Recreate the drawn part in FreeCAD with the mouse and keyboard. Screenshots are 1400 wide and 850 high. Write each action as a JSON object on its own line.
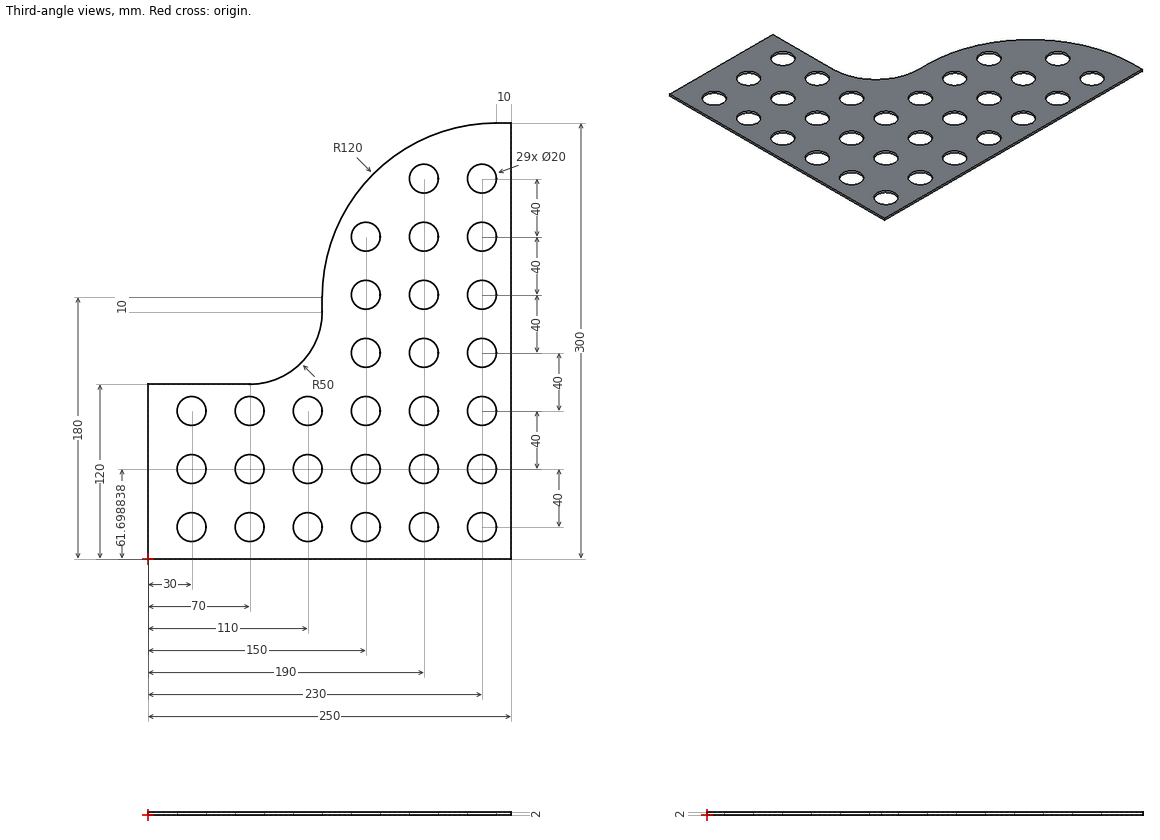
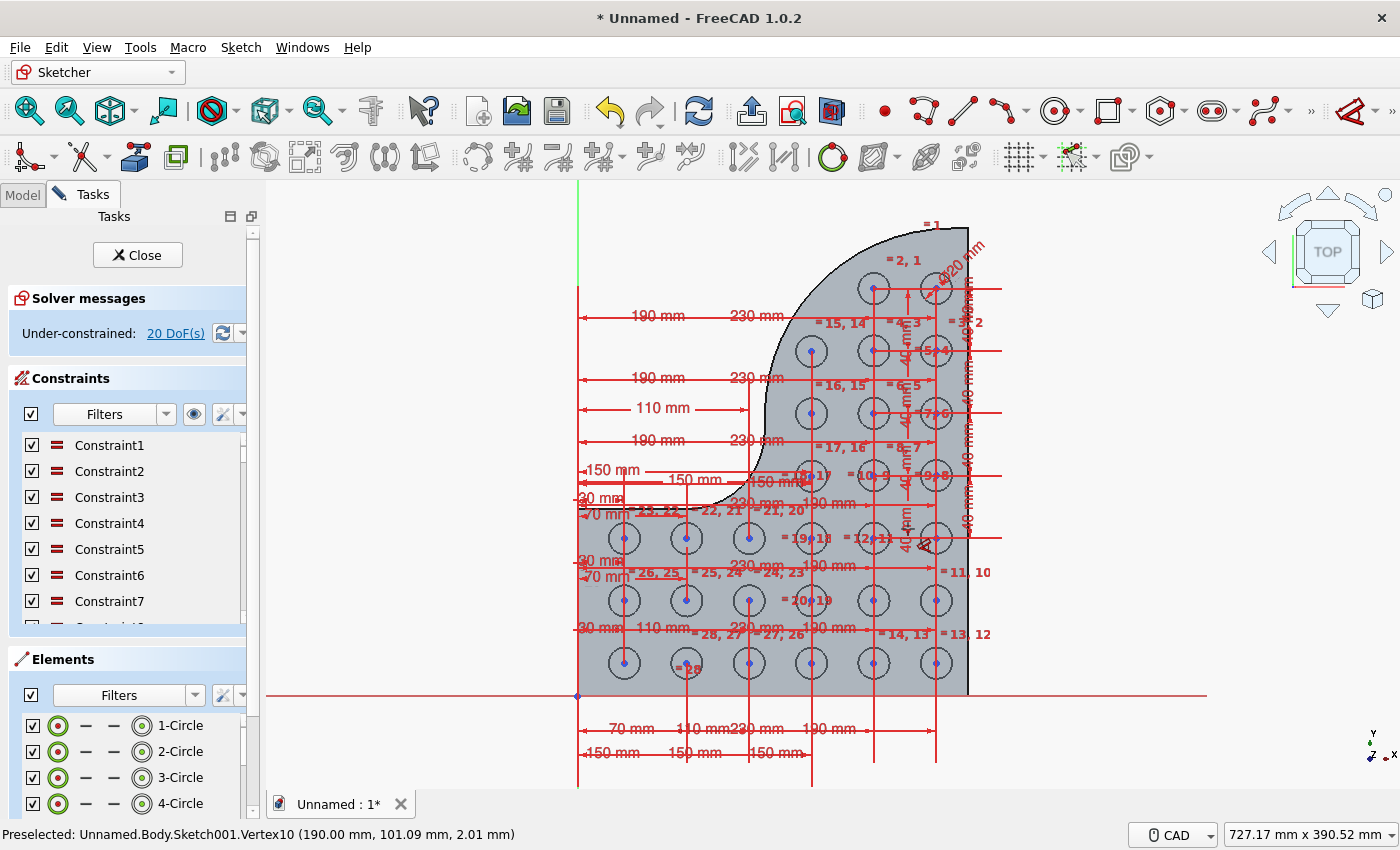
{"action": "left_click", "coordinate": [936, 538]}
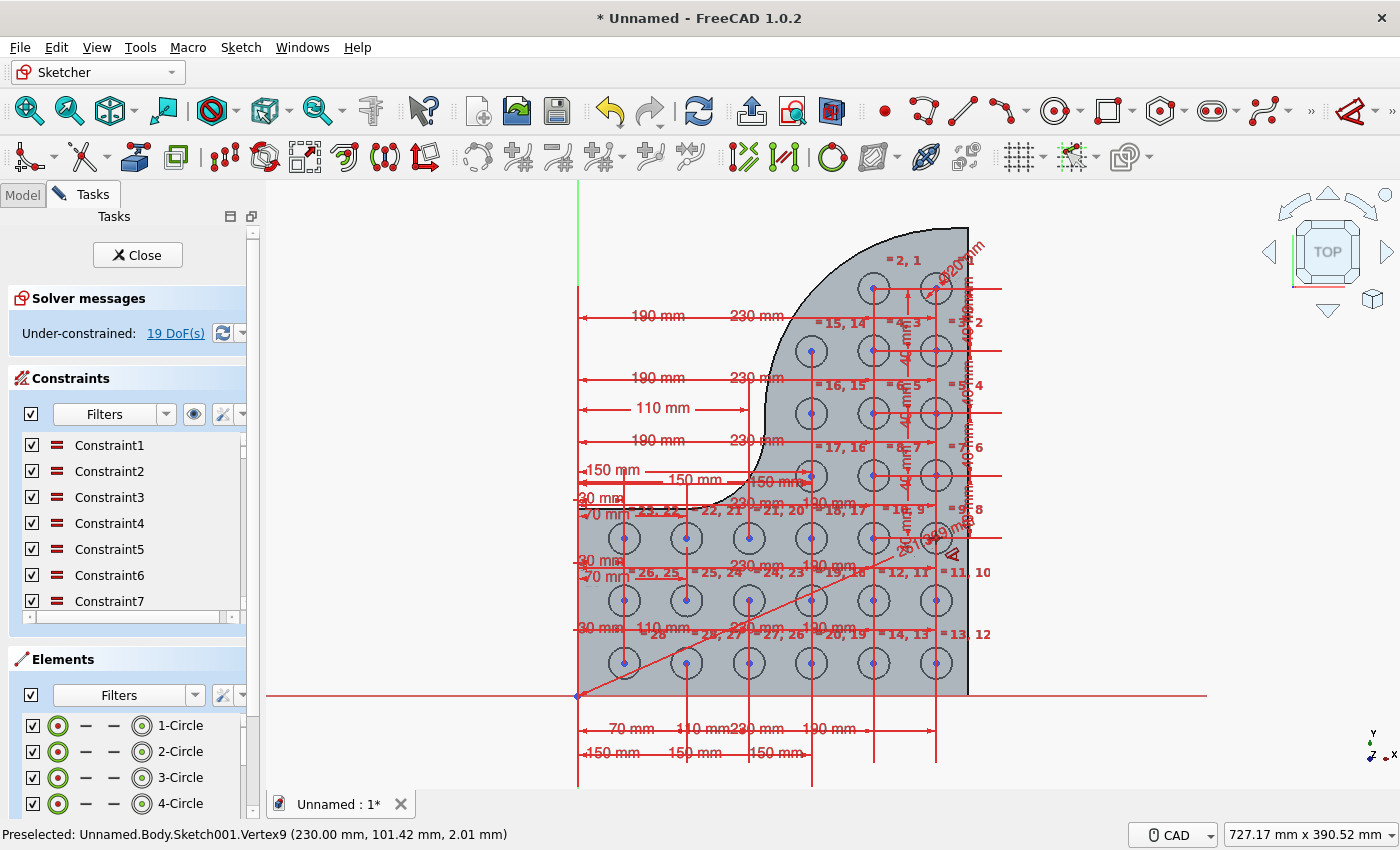
{"action": "left_click", "coordinate": [936, 601]}
{"action": "left_click", "coordinate": [970, 570]}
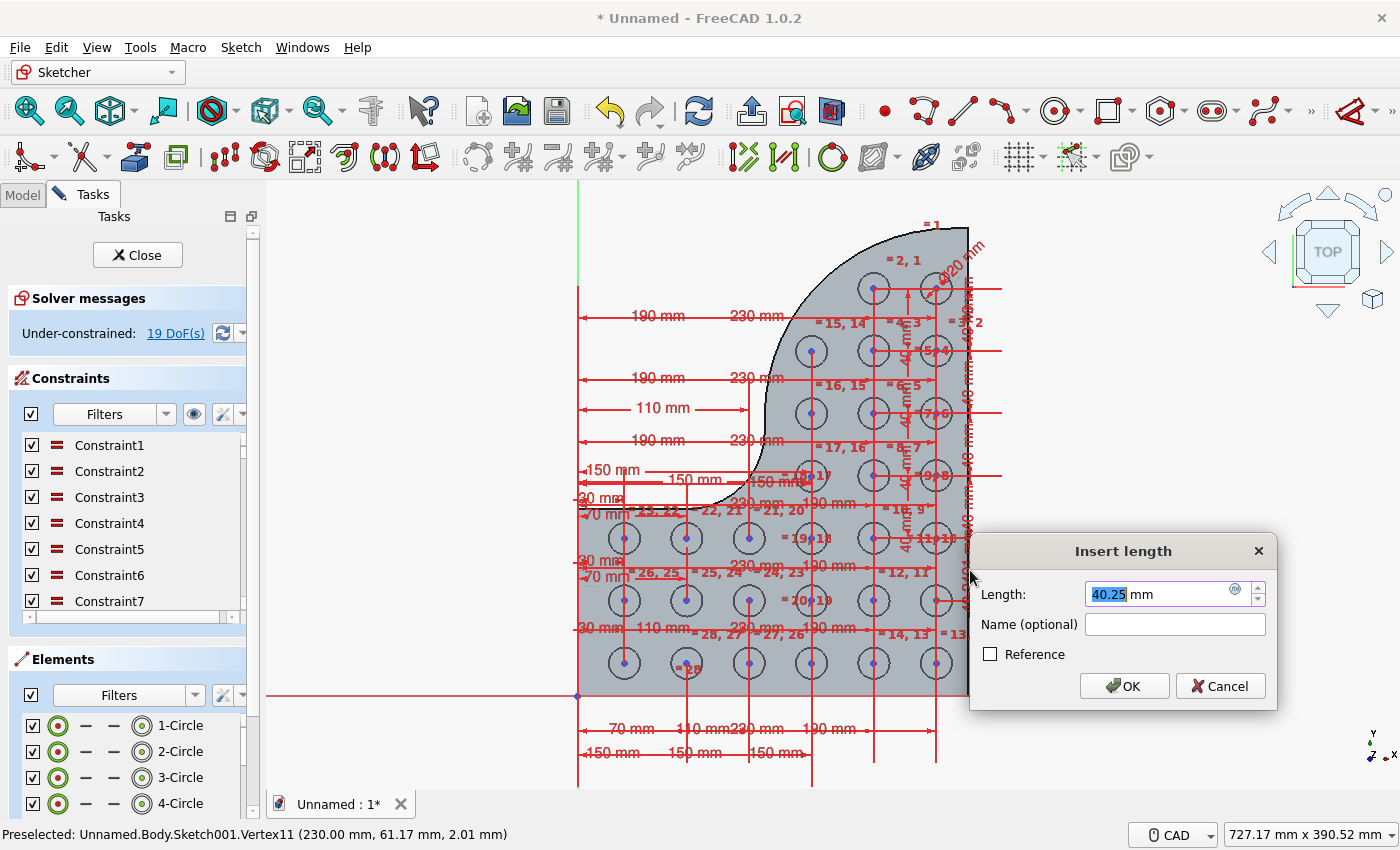
{"action": "type", "text": "40"}
{"action": "key", "text": "Return"}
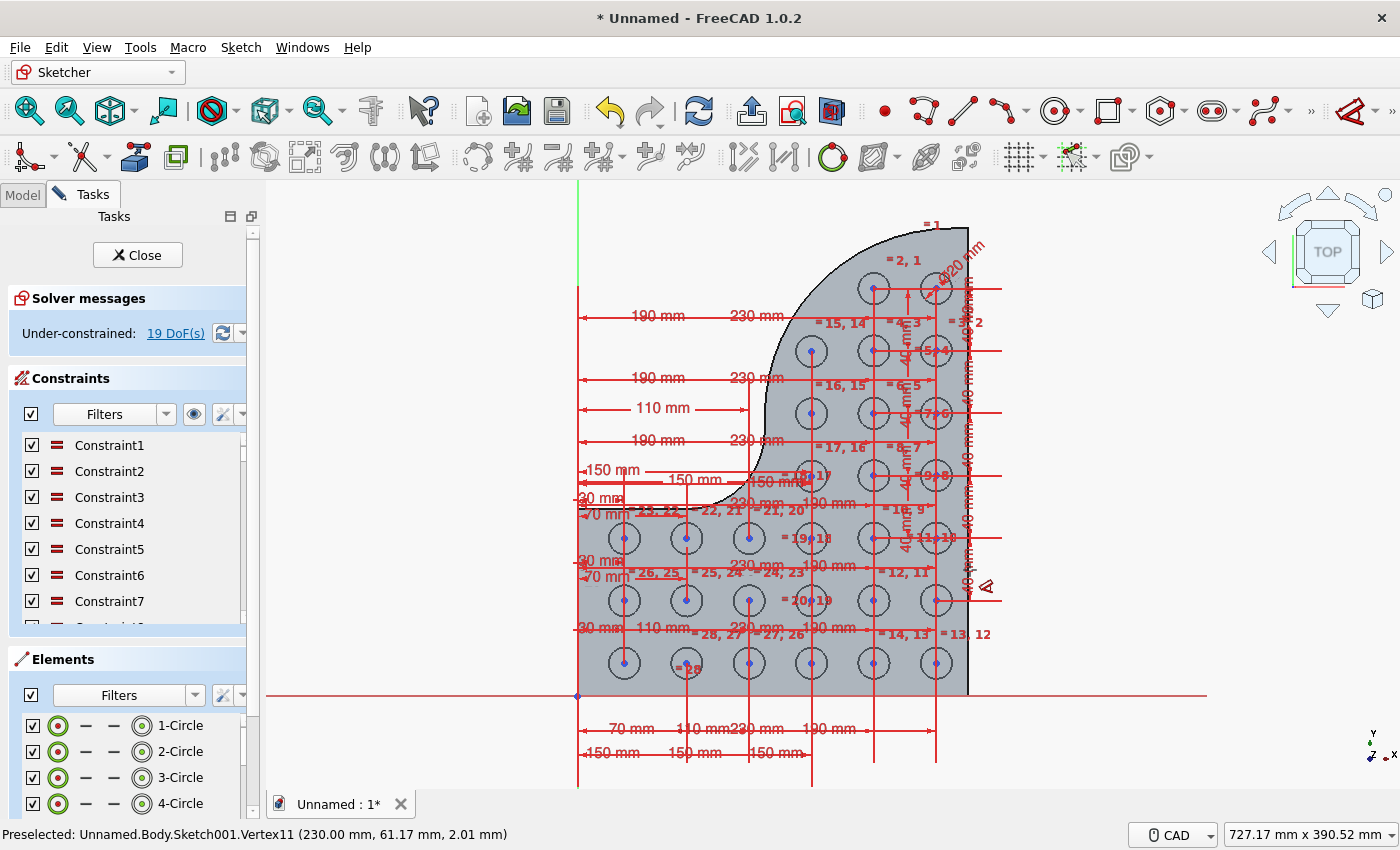
{"action": "left_click", "coordinate": [874, 538]}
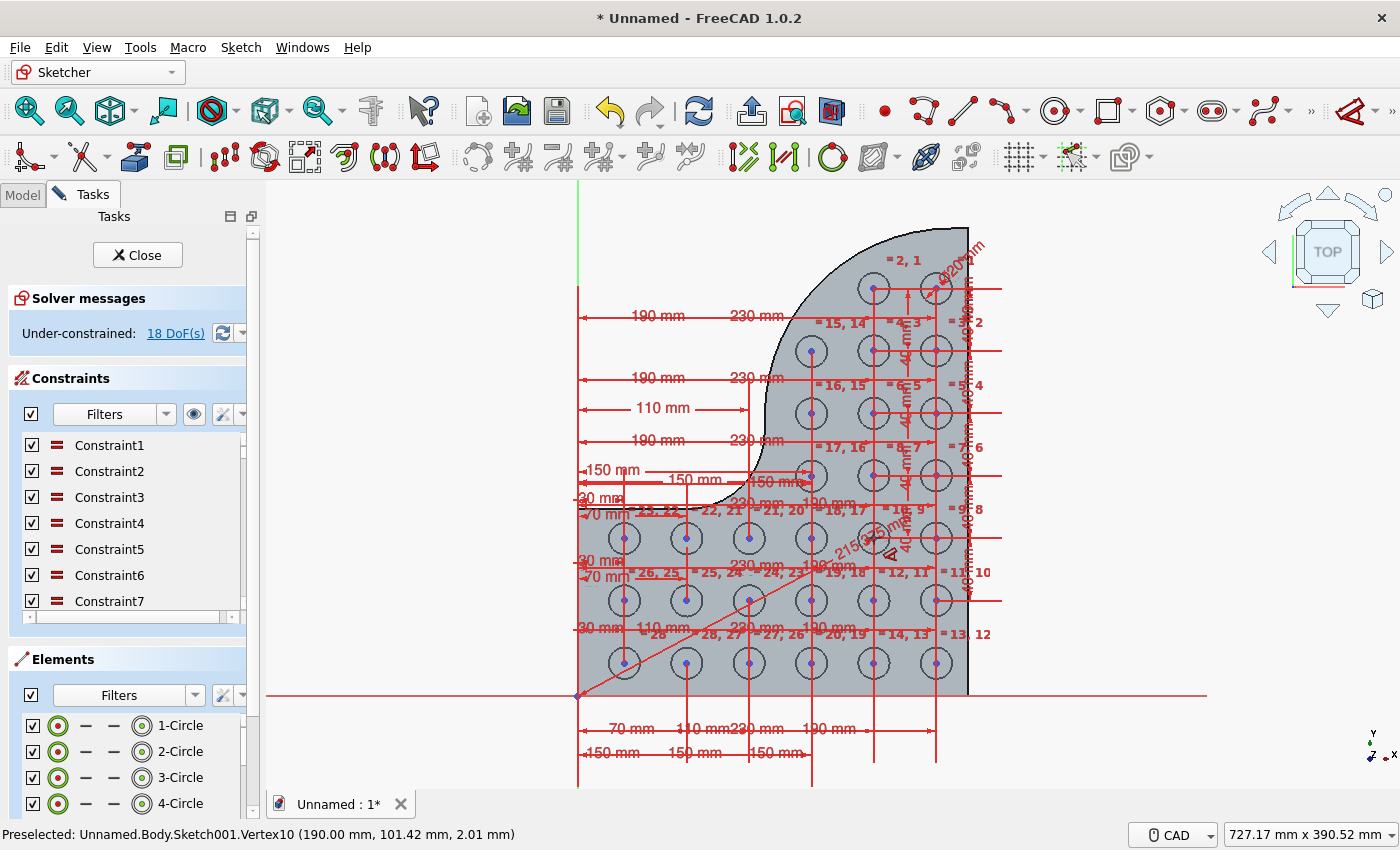
{"action": "left_click", "coordinate": [874, 601]}
{"action": "left_click", "coordinate": [908, 591]}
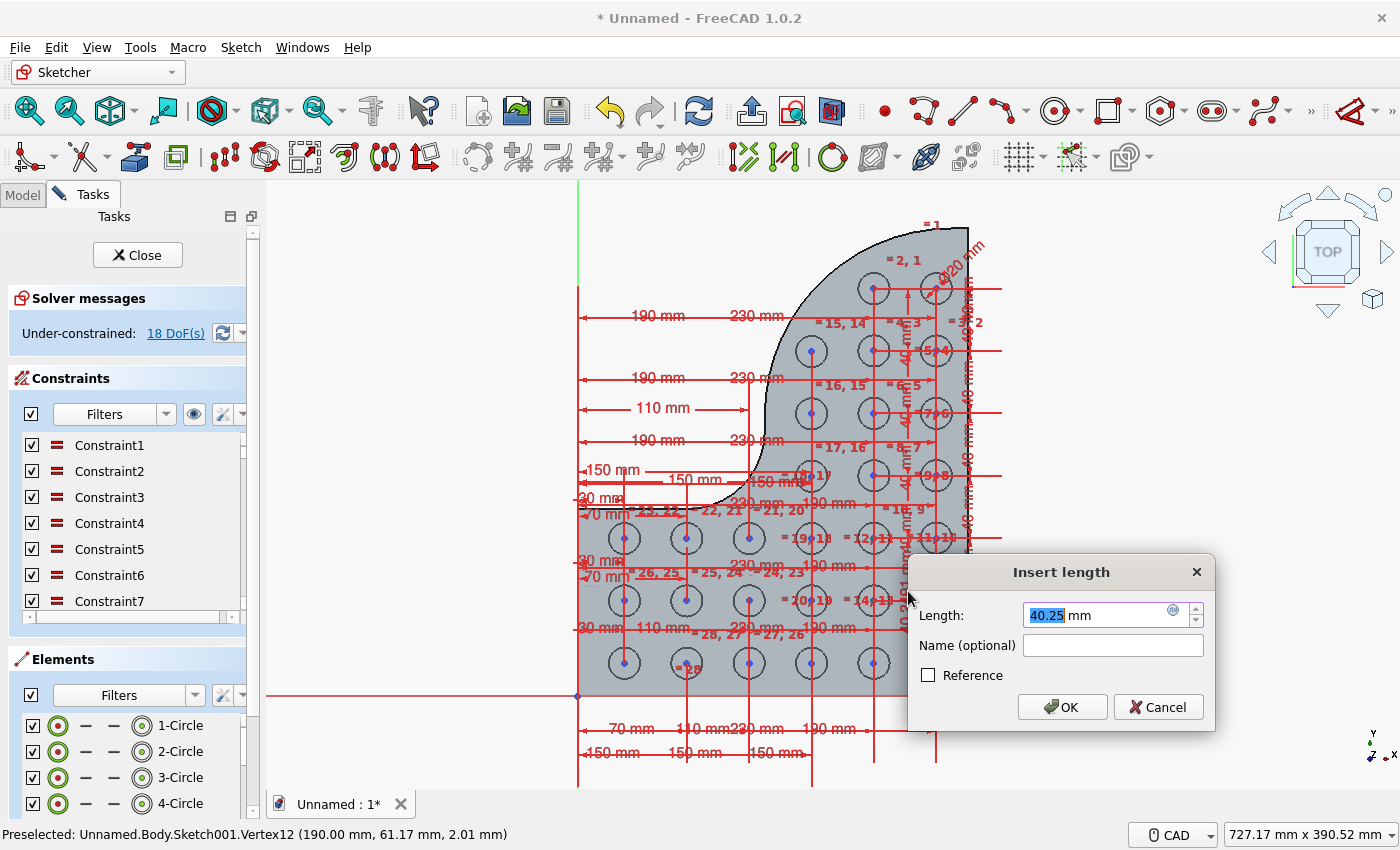
{"action": "type", "text": "40"}
{"action": "key", "text": "Return"}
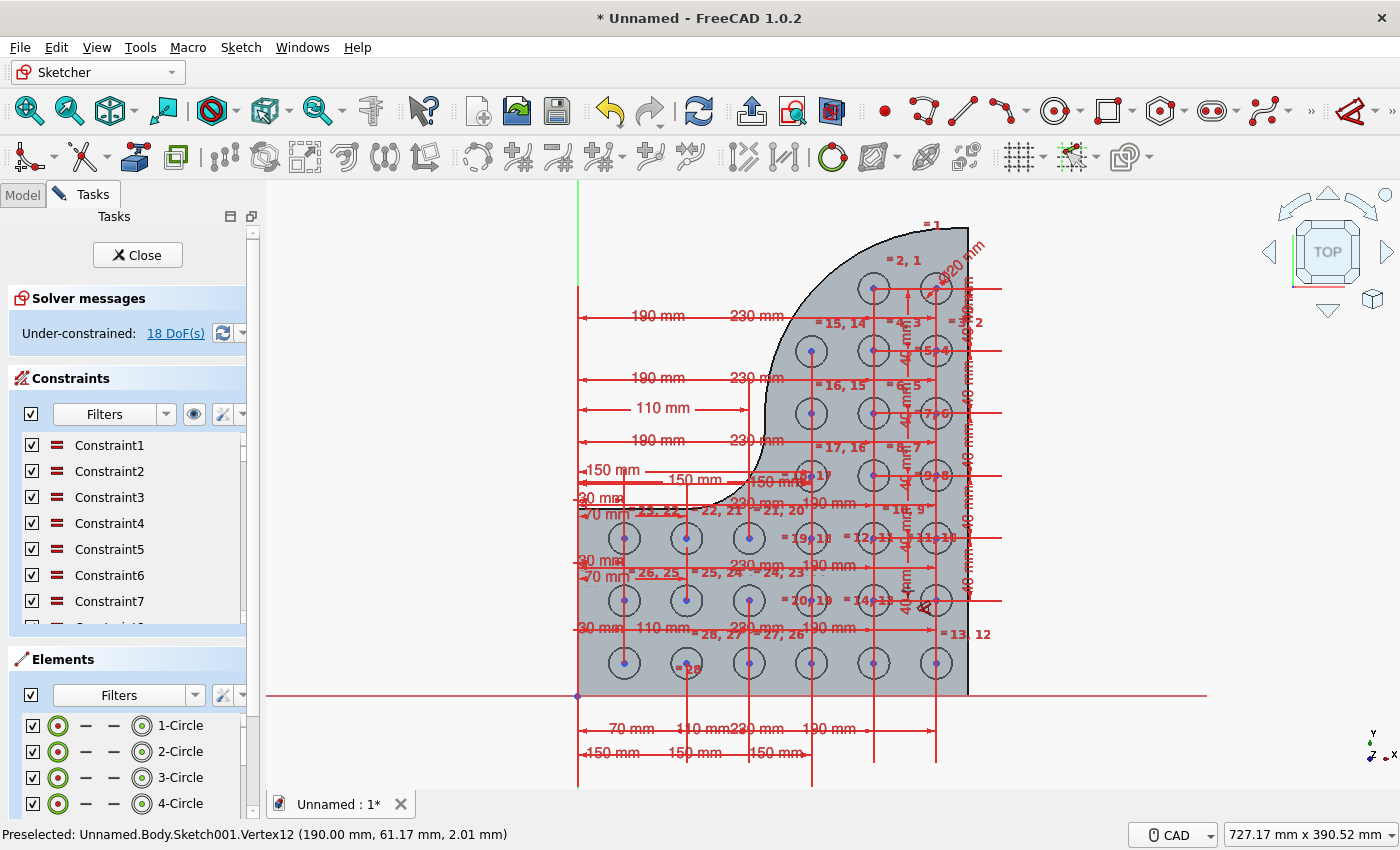
{"action": "left_click", "coordinate": [936, 601]}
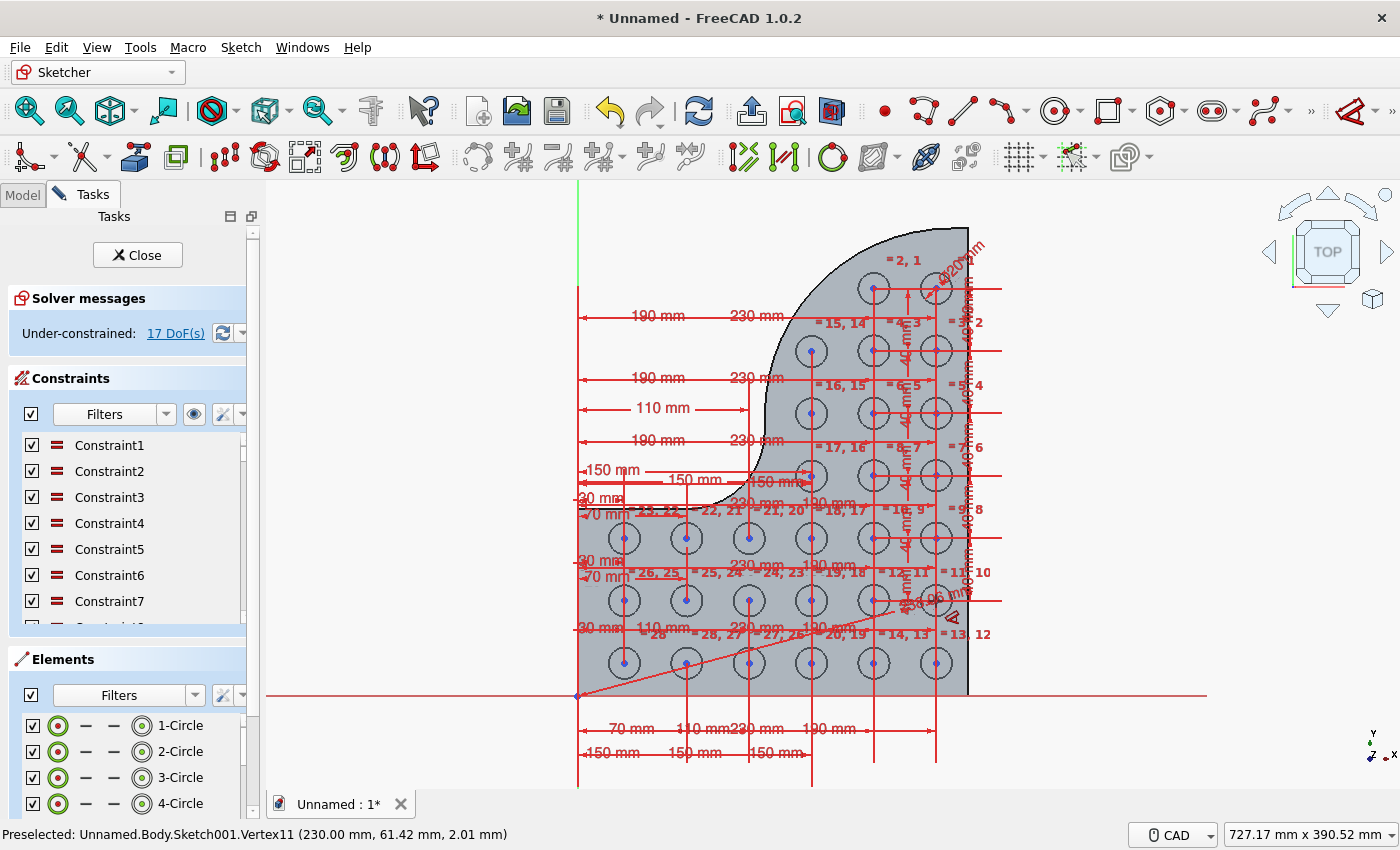
{"action": "left_click", "coordinate": [936, 663]}
{"action": "left_click", "coordinate": [970, 632]}